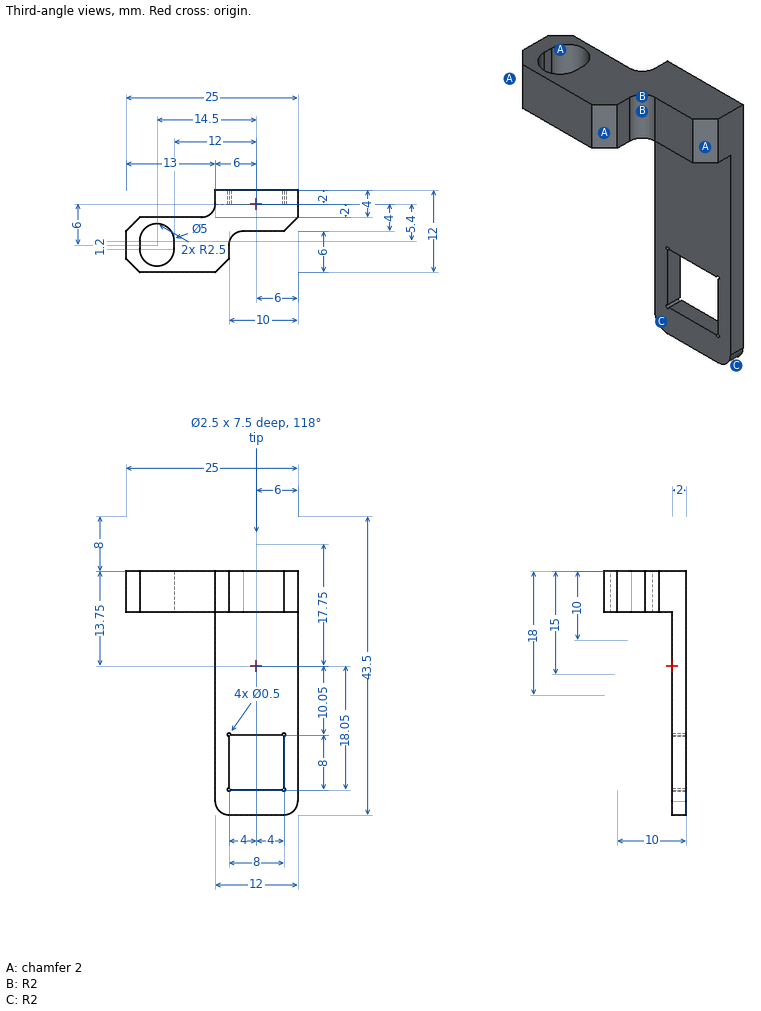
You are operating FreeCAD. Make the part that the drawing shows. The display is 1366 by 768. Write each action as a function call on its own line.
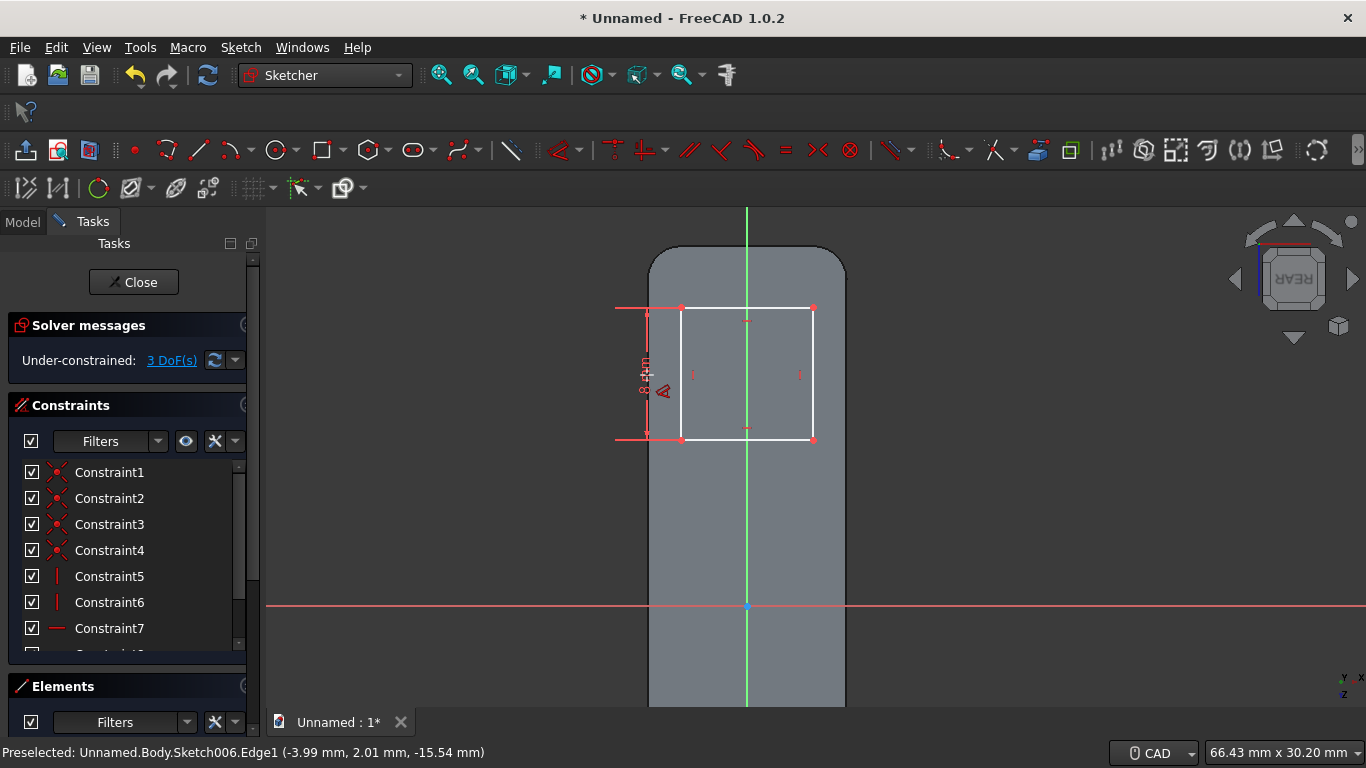
click(721, 440)
click(717, 406)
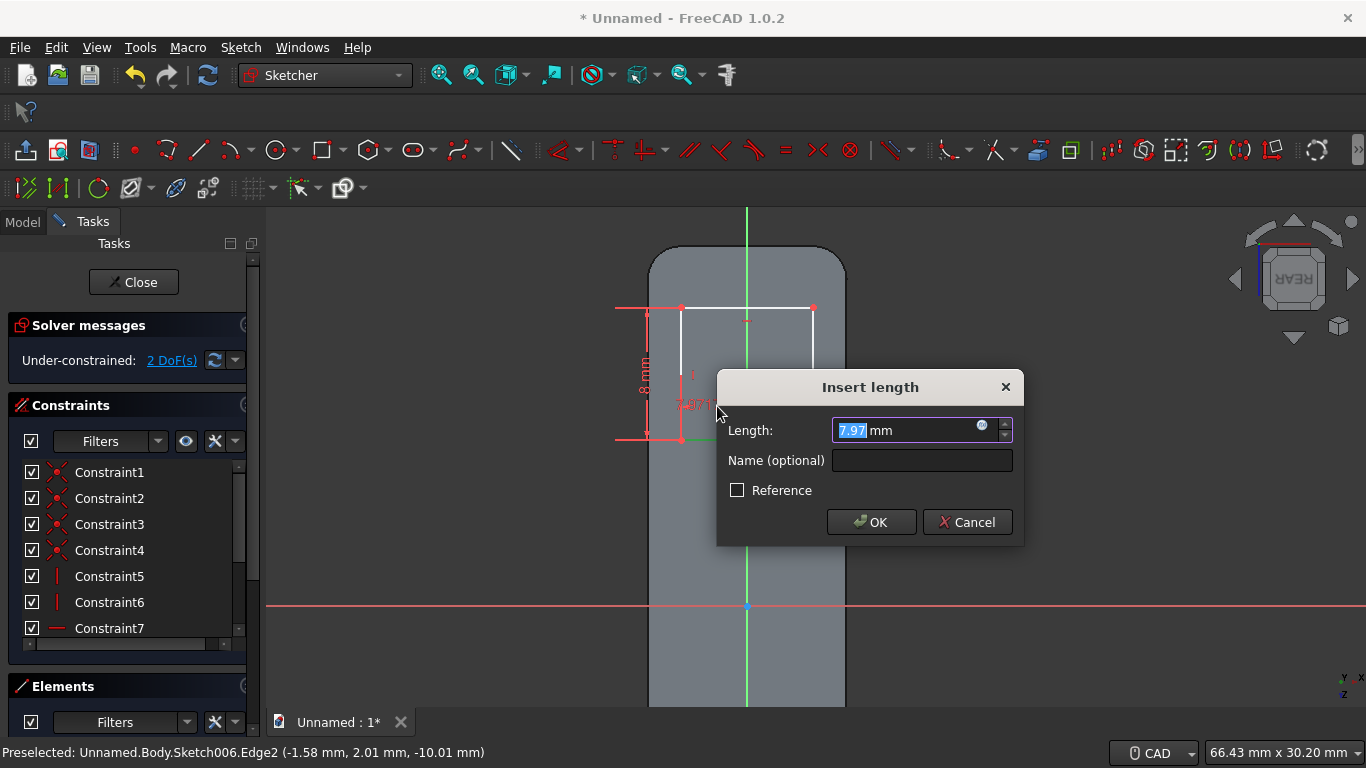
text(8)
key(Return)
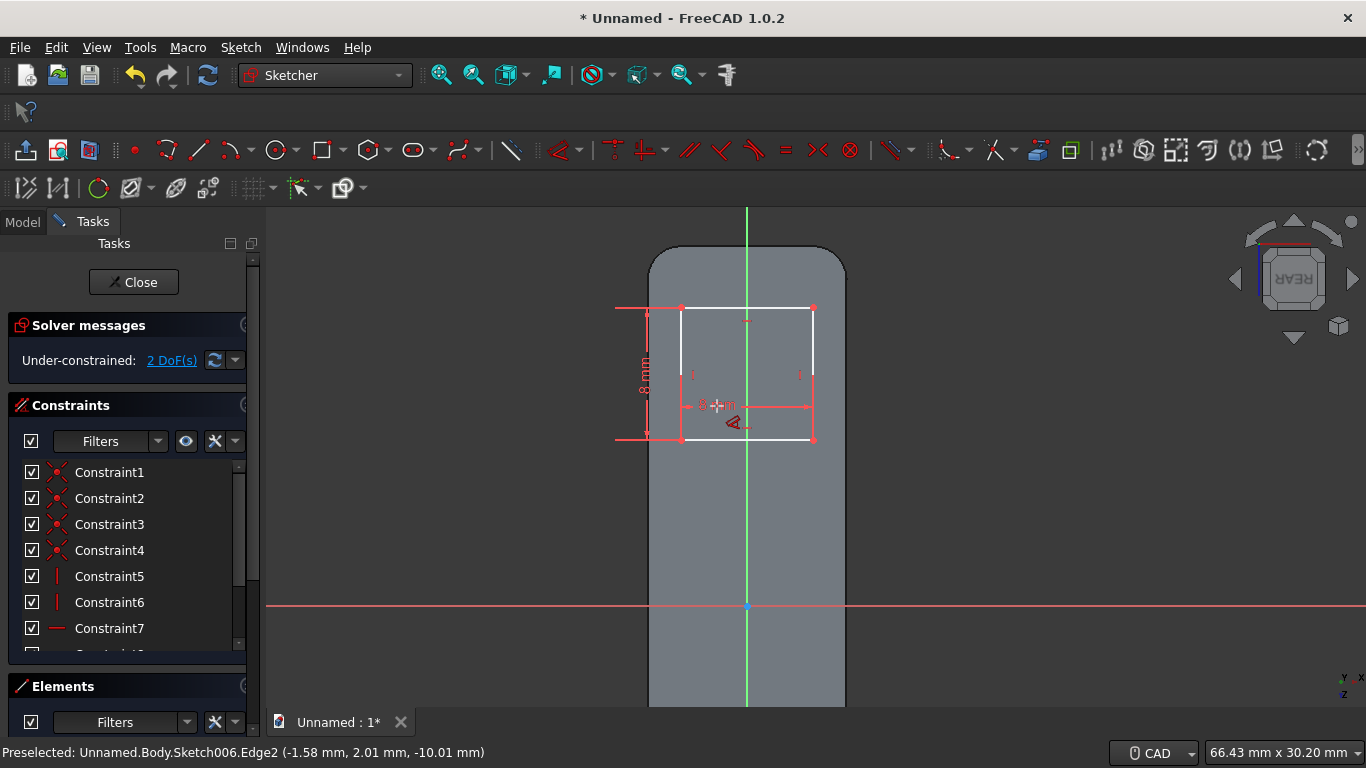
click(681, 308)
click(714, 640)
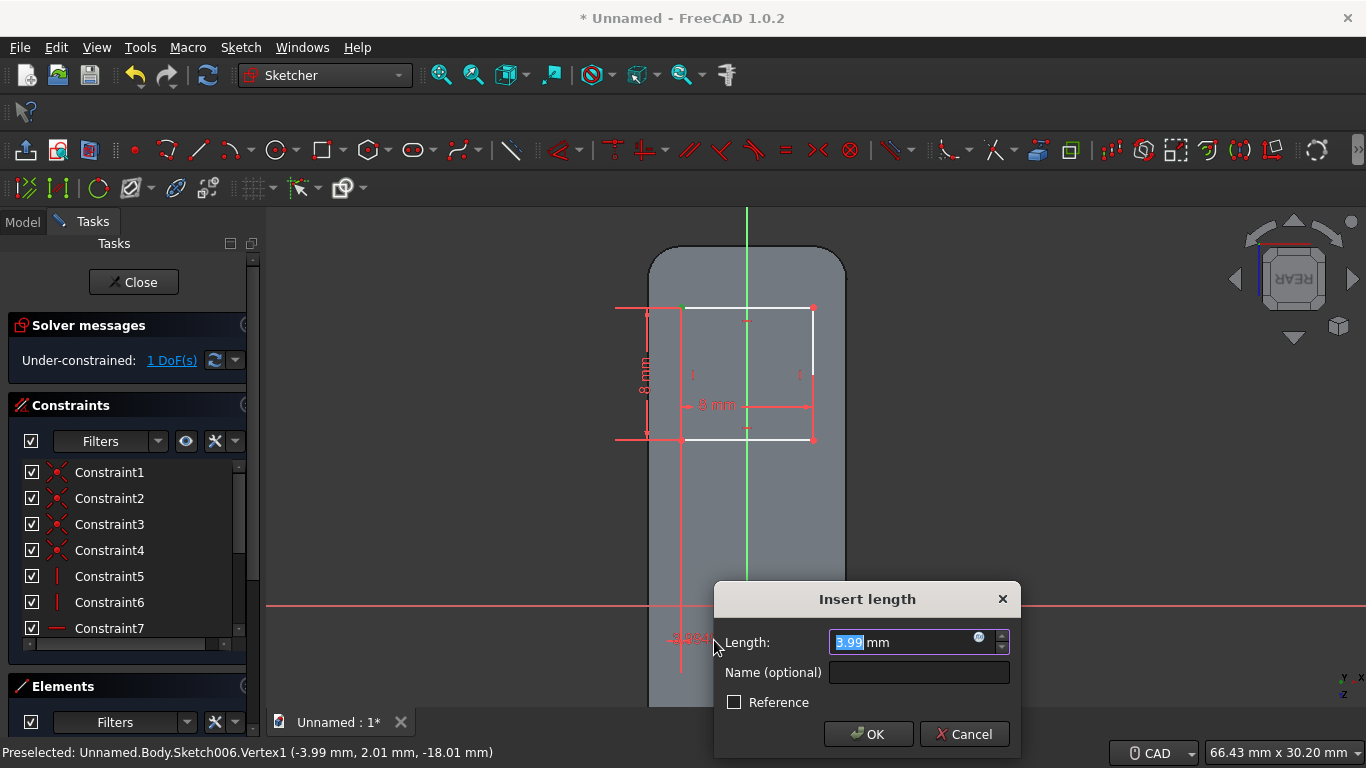
text(4)
key(Return)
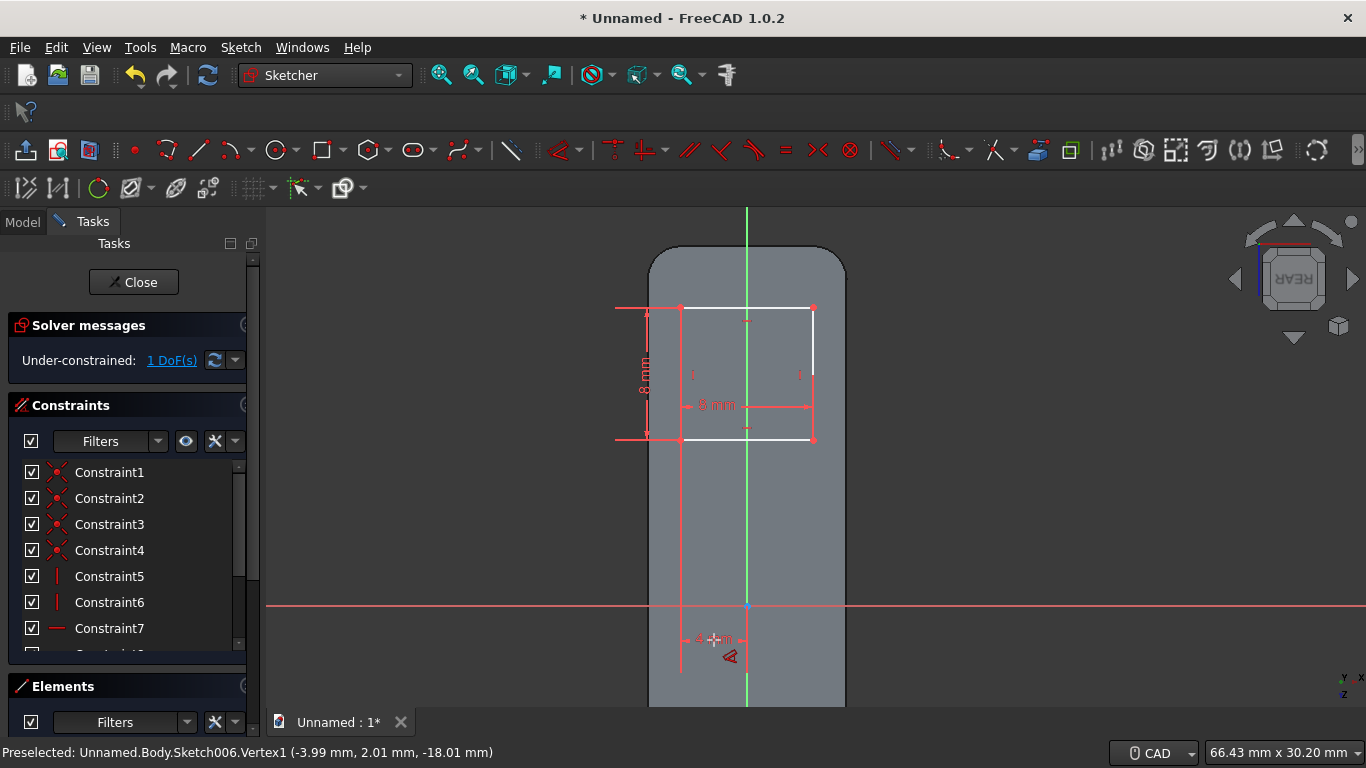
click(681, 308)
click(647, 457)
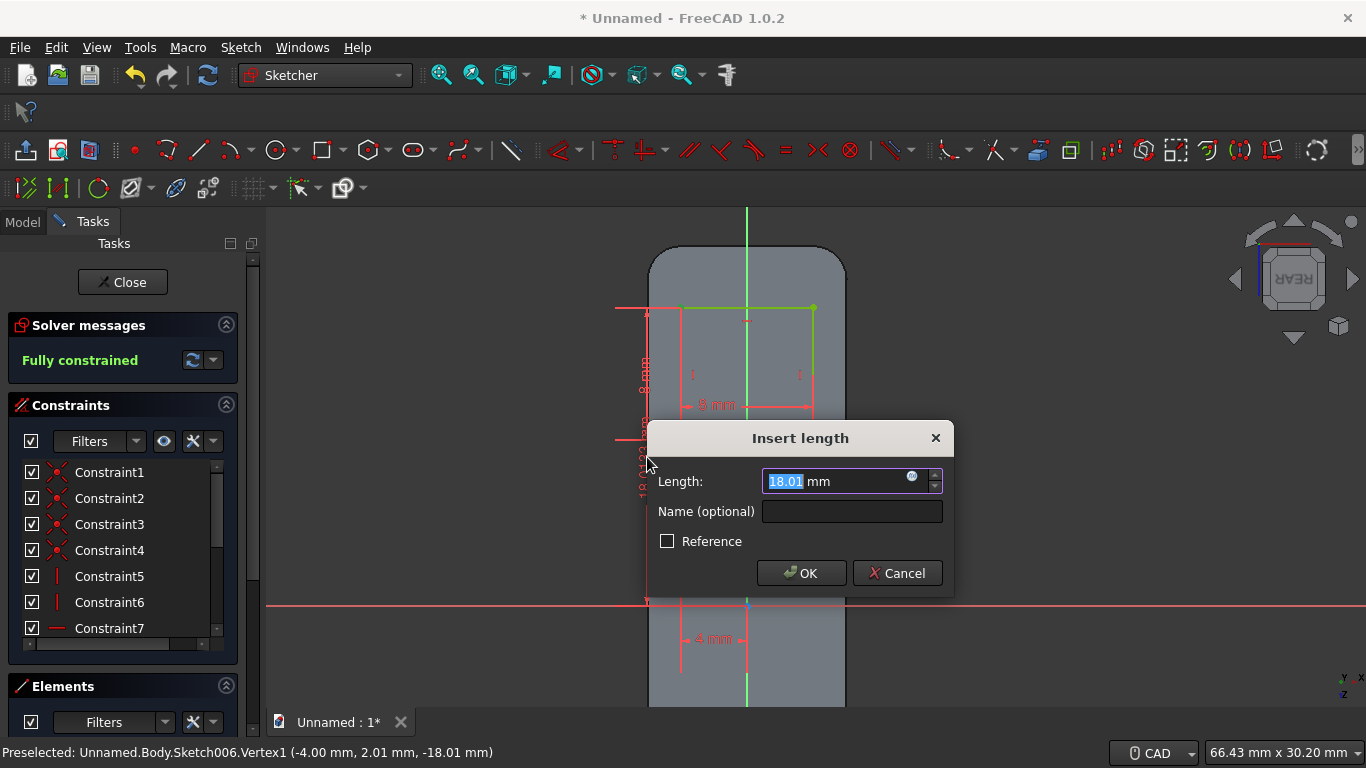
text(18.05)
key(Return)
key(Escape)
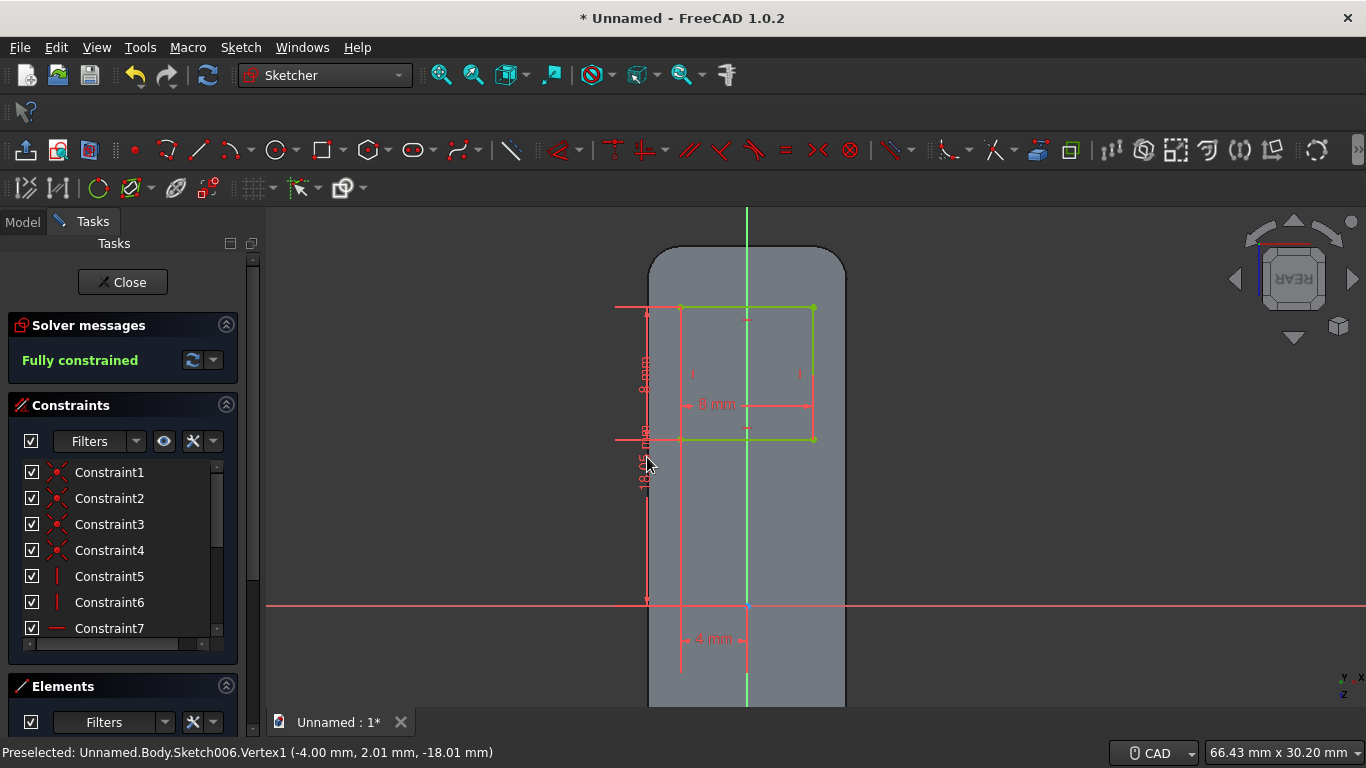
click(123, 282)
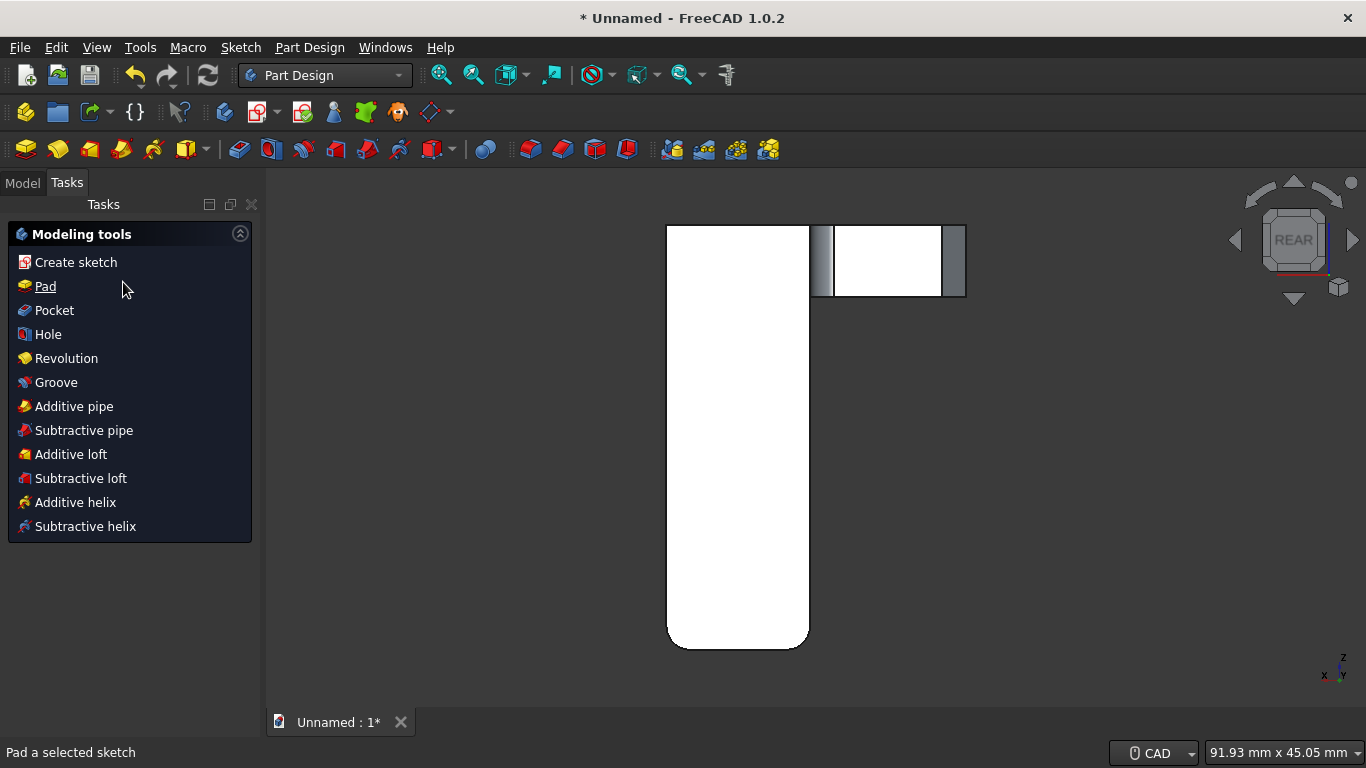
click(240, 150)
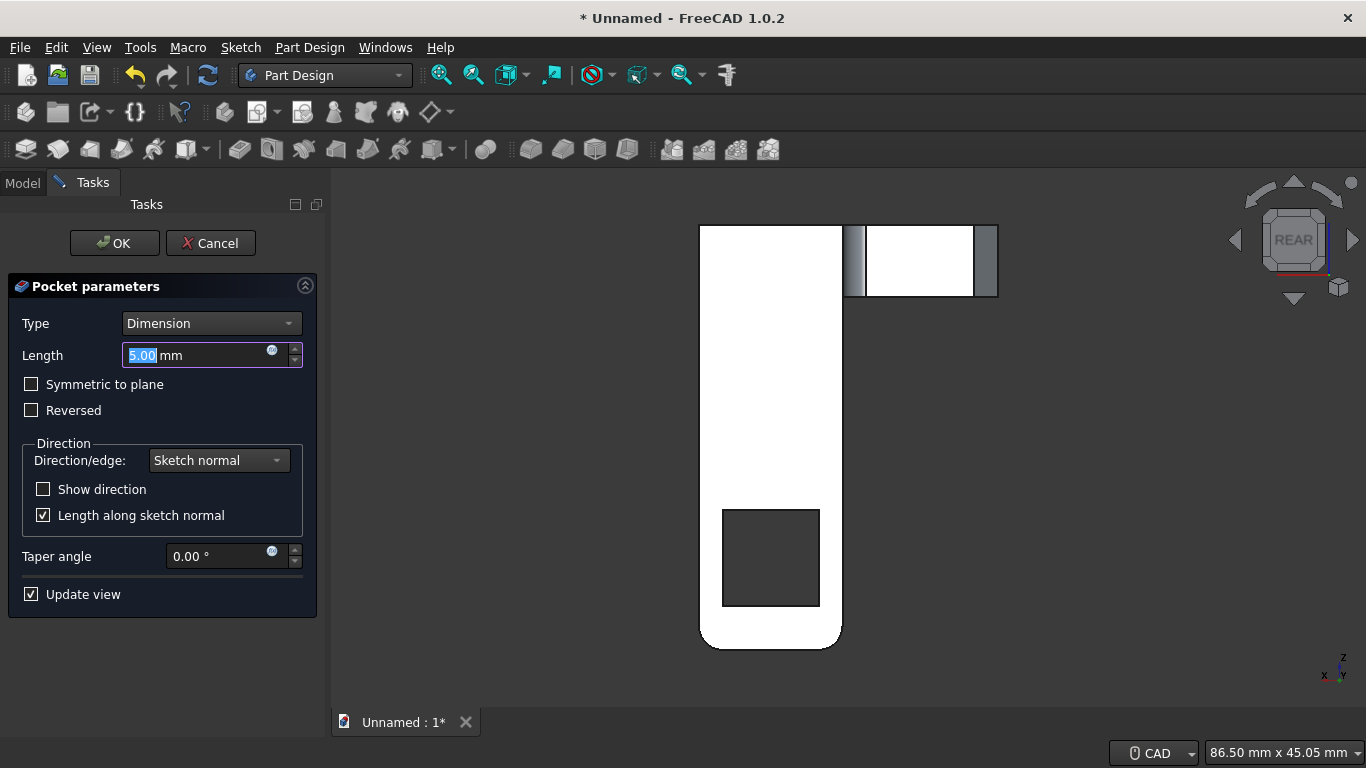
text(10)
key(Tab)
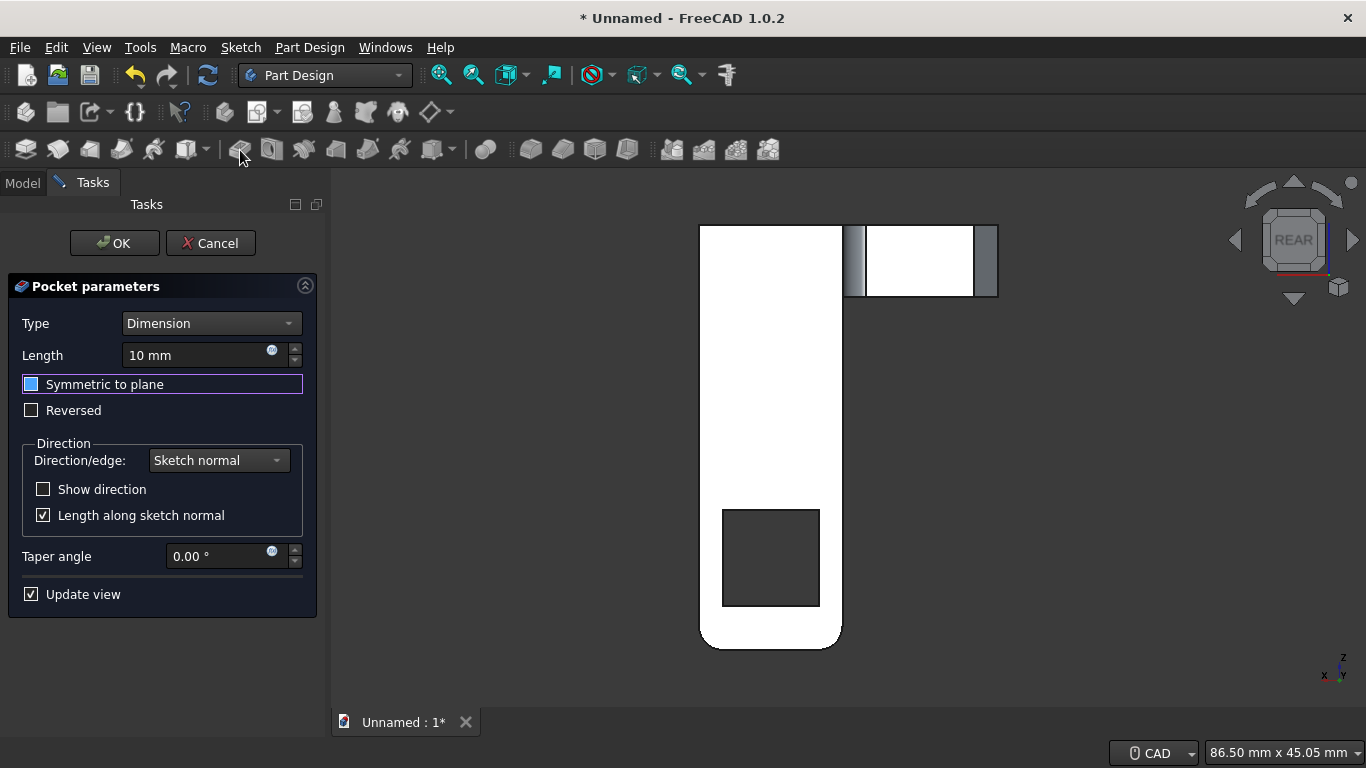
click(115, 243)